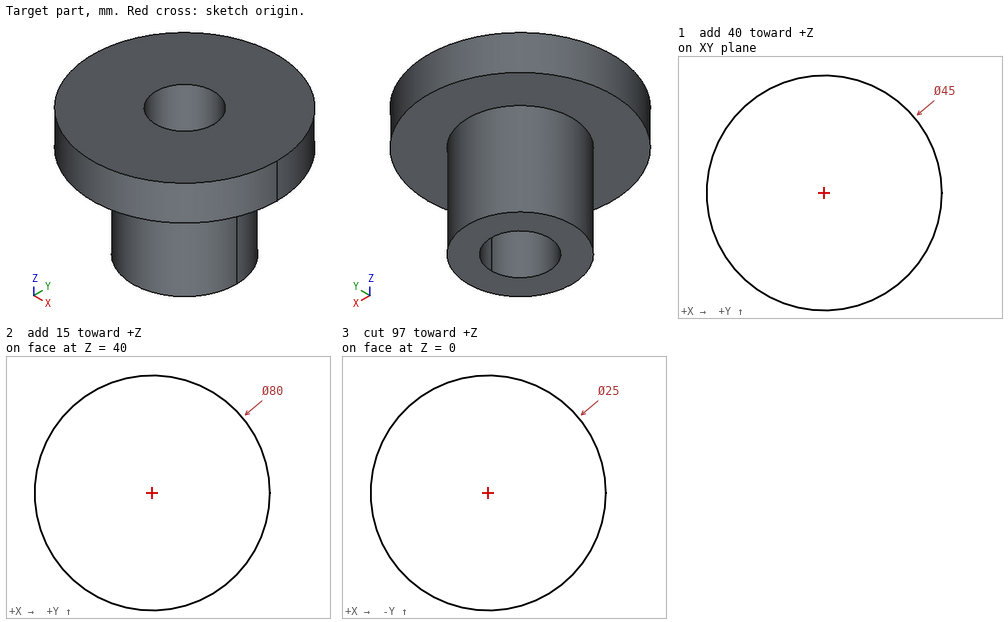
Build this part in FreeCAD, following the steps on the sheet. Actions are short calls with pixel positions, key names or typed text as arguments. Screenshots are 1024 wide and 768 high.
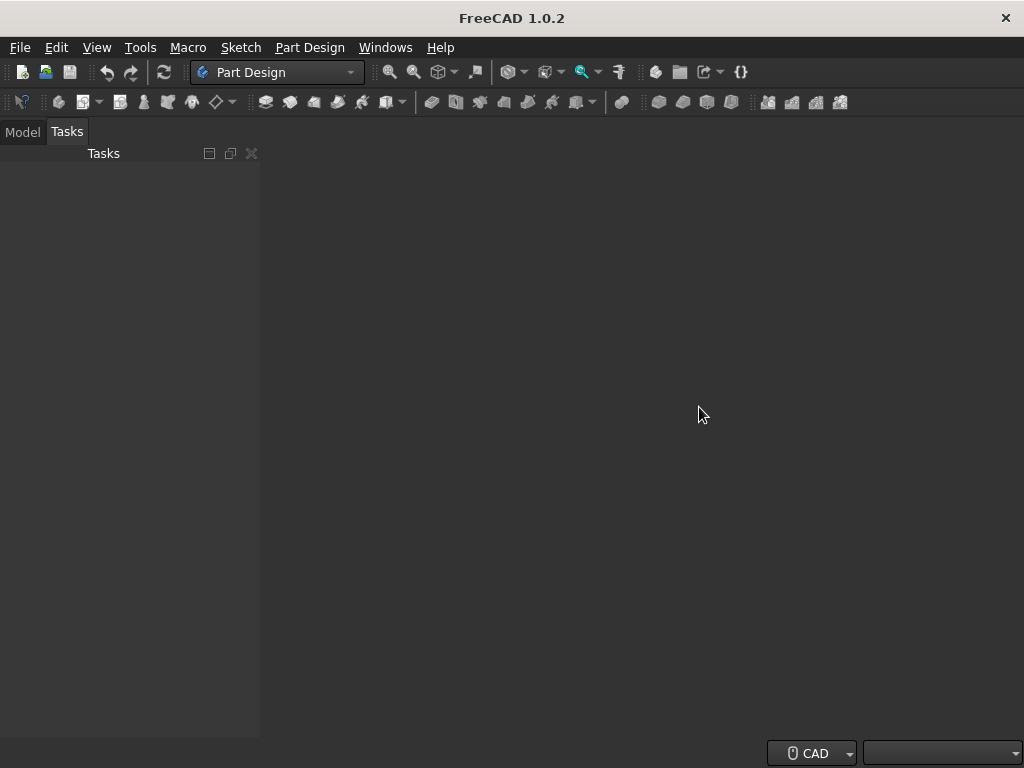
click(22, 72)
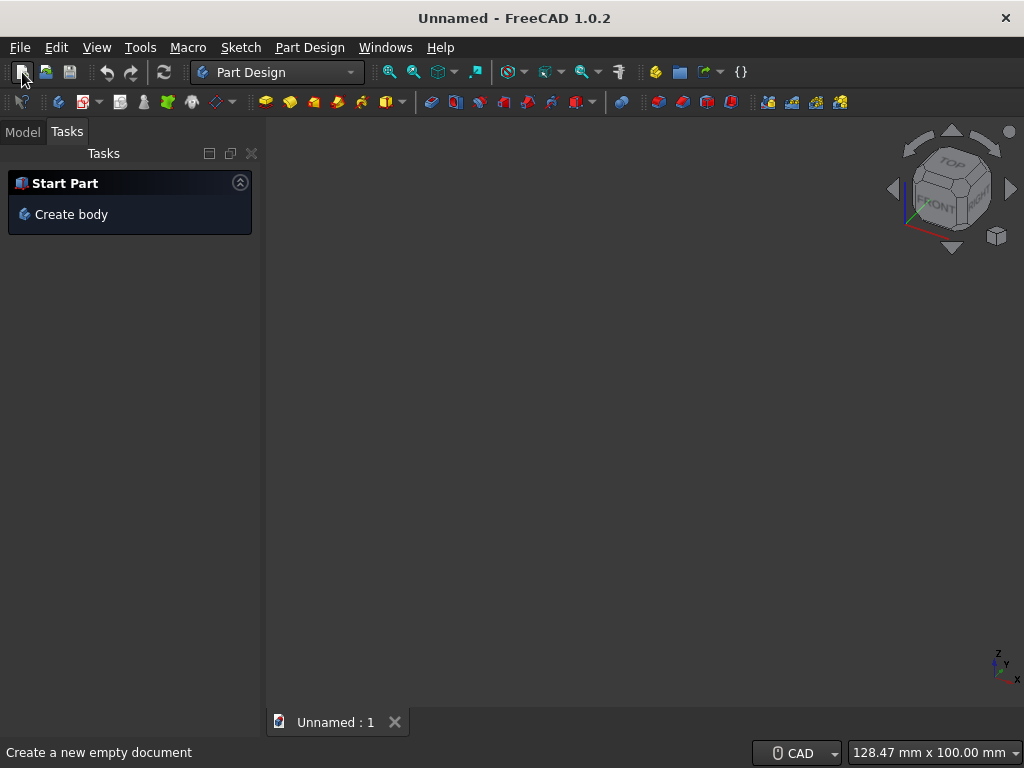
click(84, 102)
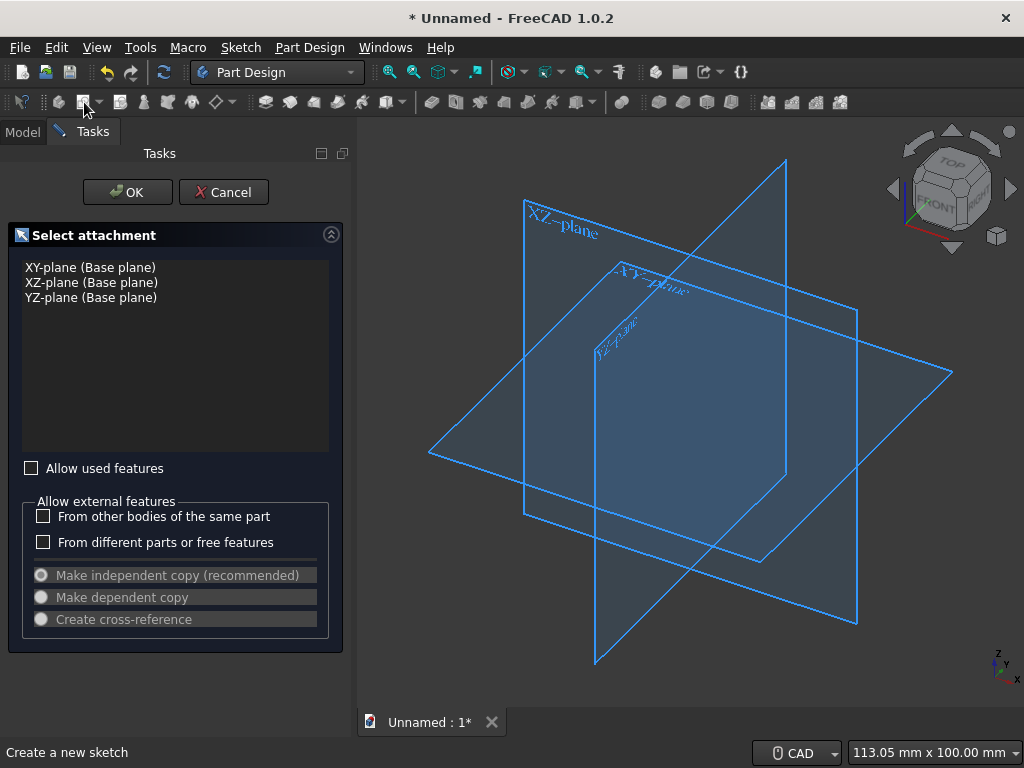
click(82, 268)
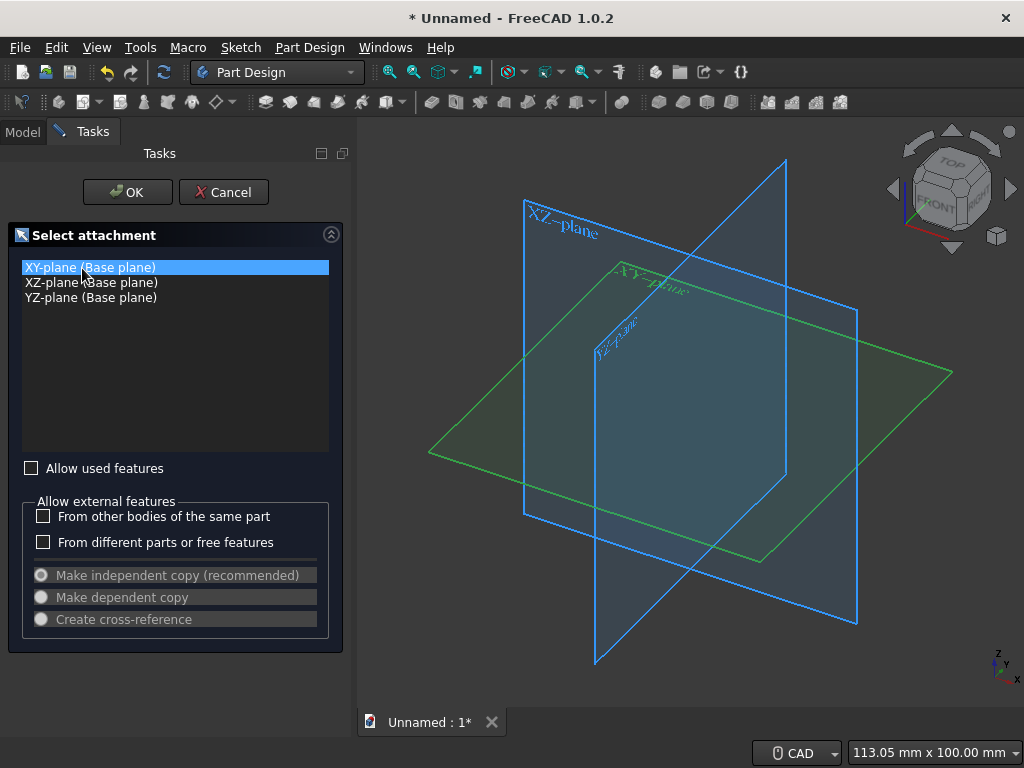
click(128, 192)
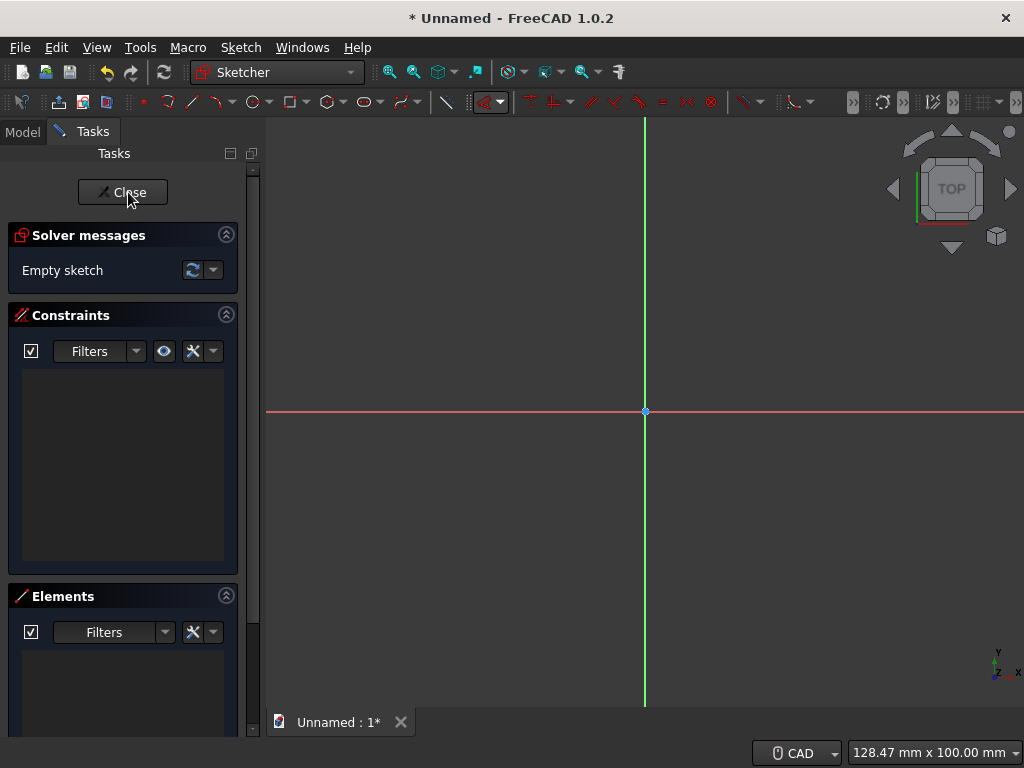
scroll(784, 412, up, 2)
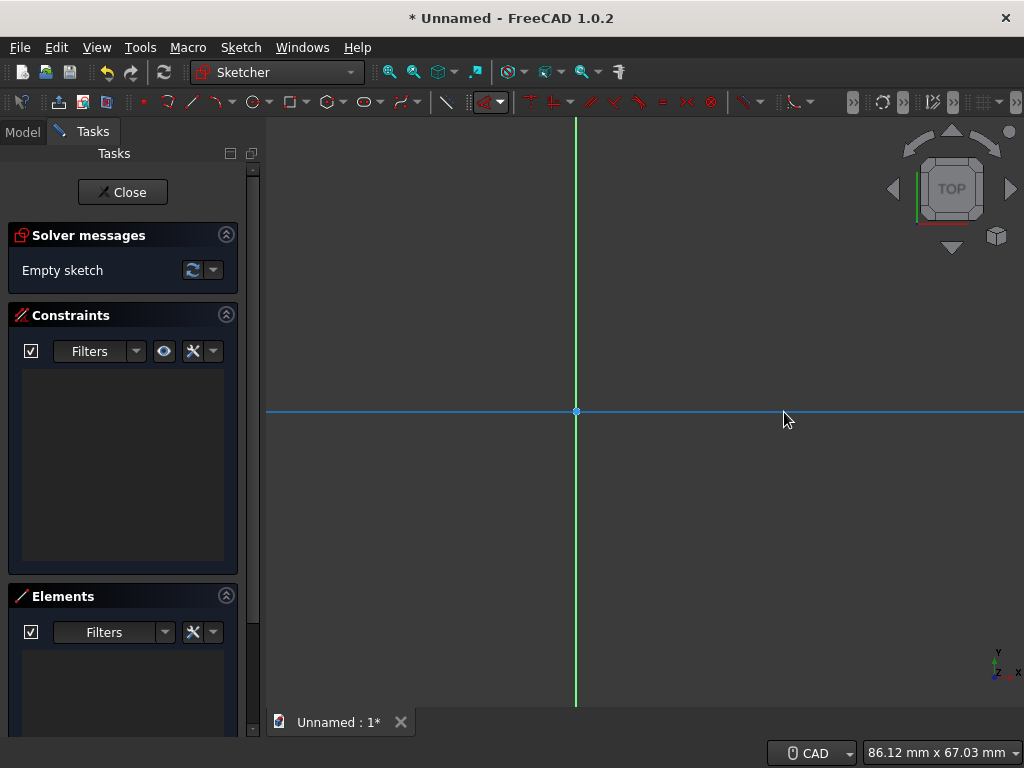
click(254, 102)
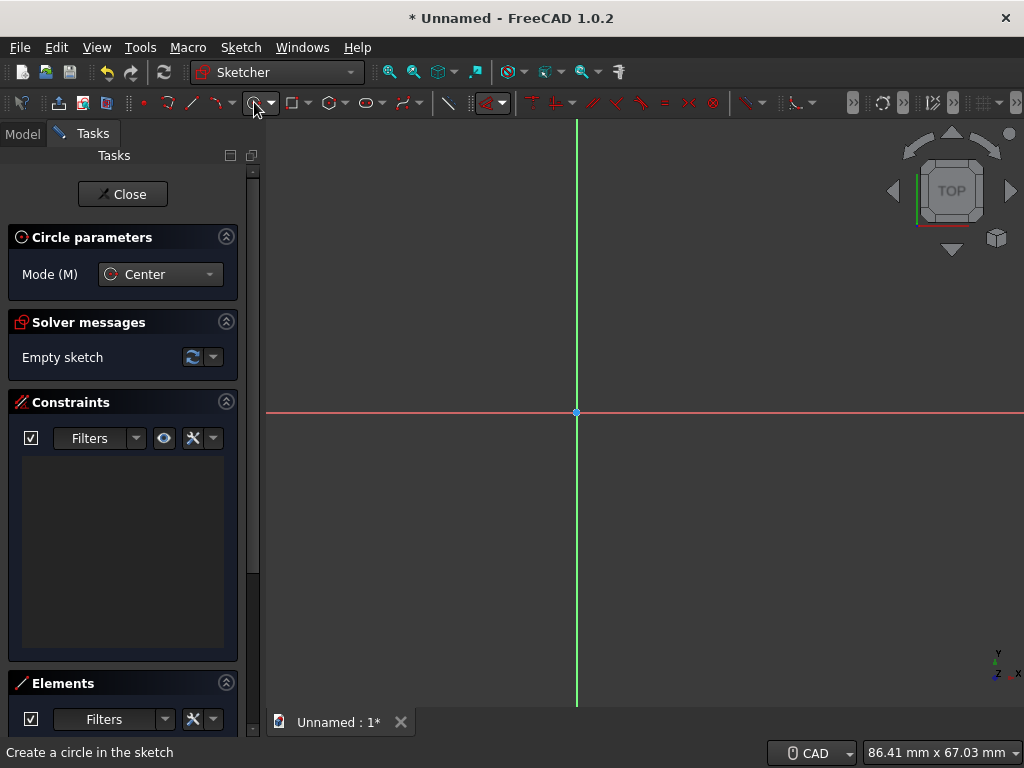
click(577, 413)
click(716, 273)
key(Escape)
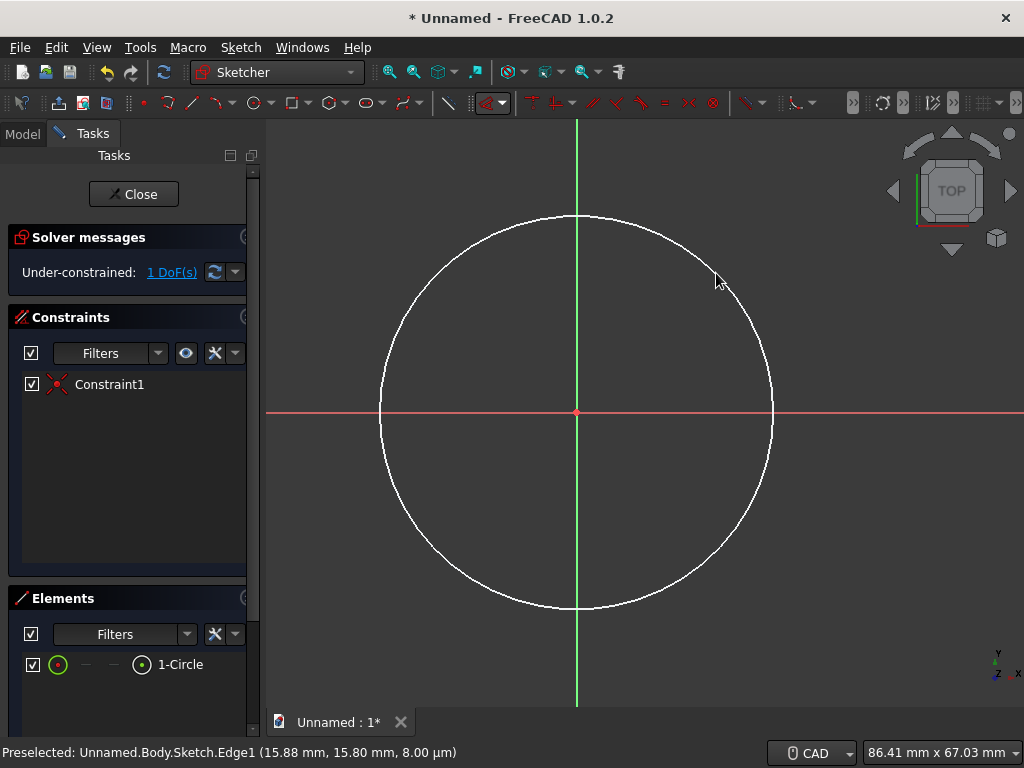
click(486, 104)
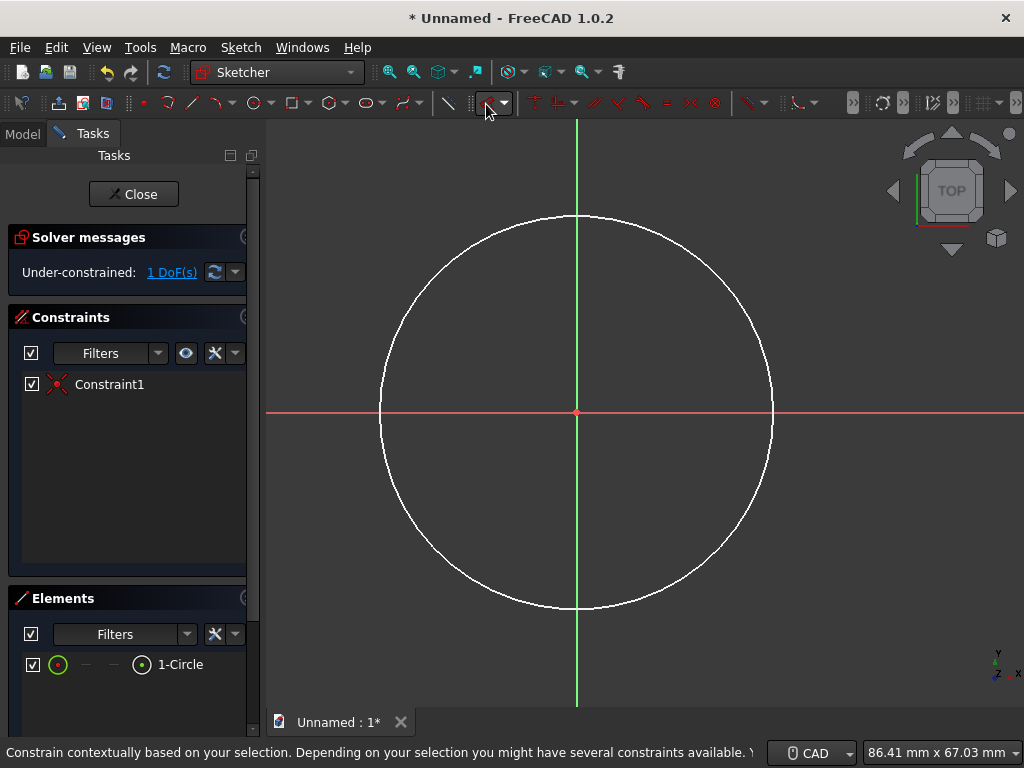
click(715, 273)
click(738, 250)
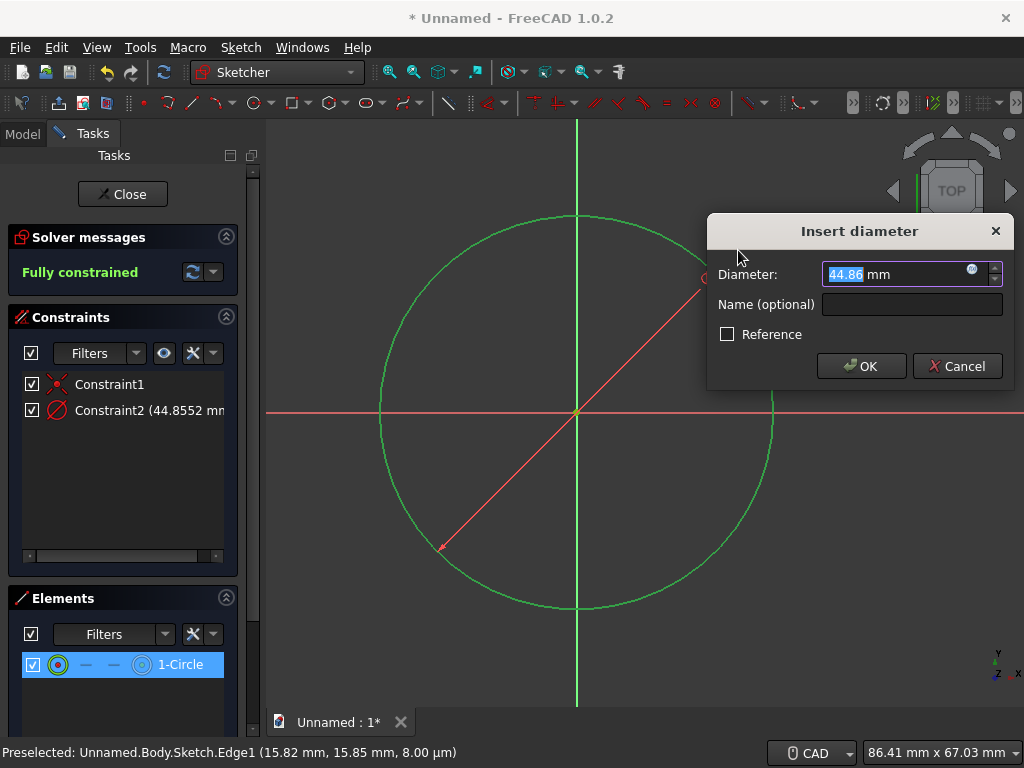
text(45)
key(Return)
key(Escape)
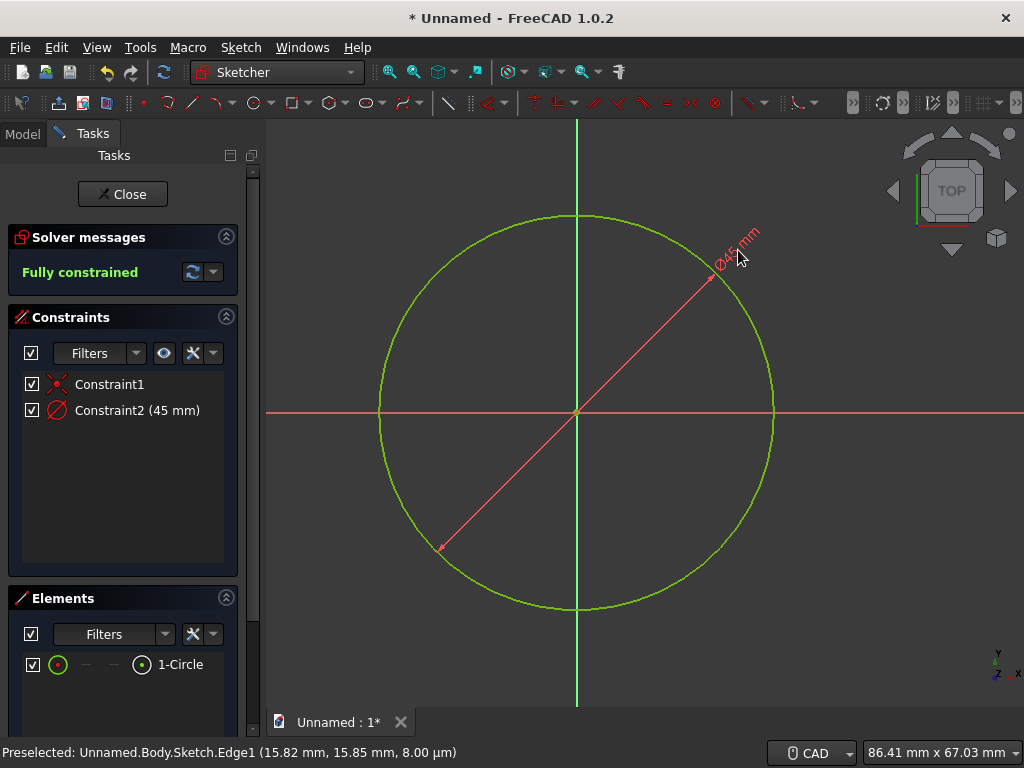
click(123, 194)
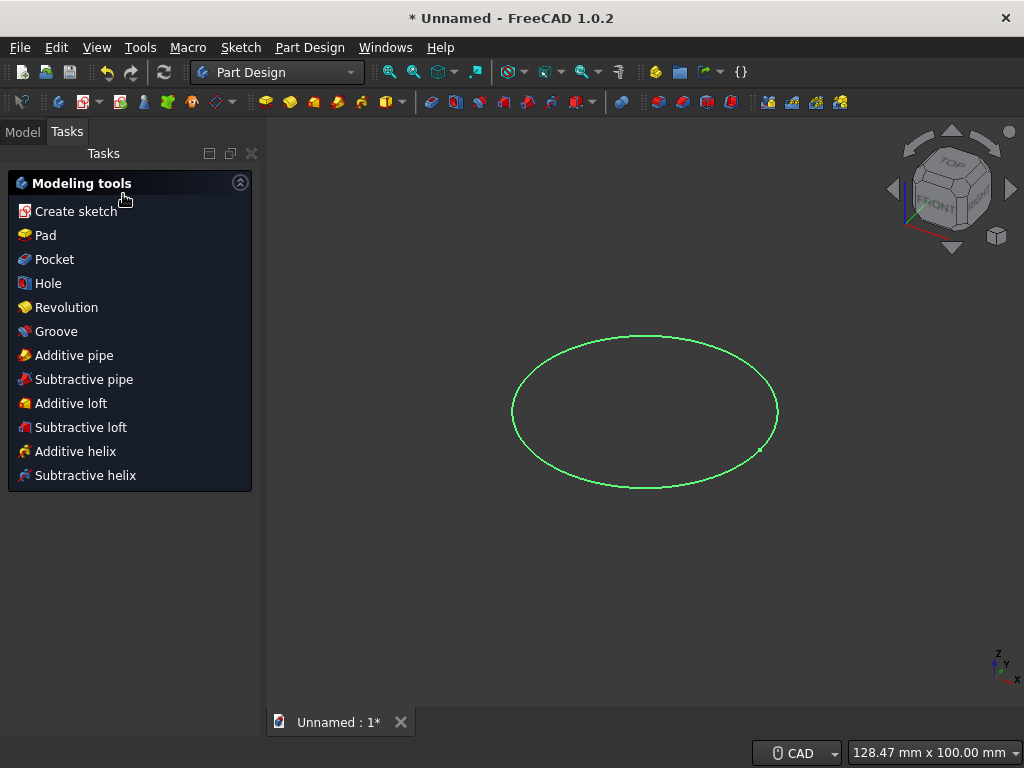
click(266, 102)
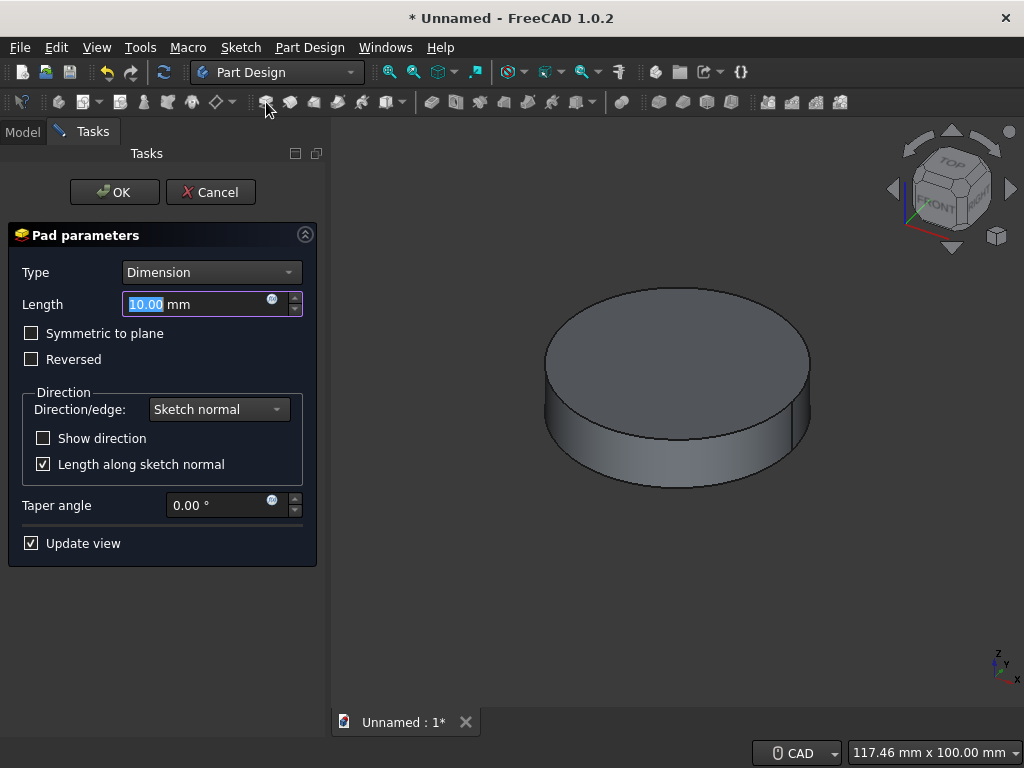
text(40)
key(Tab)